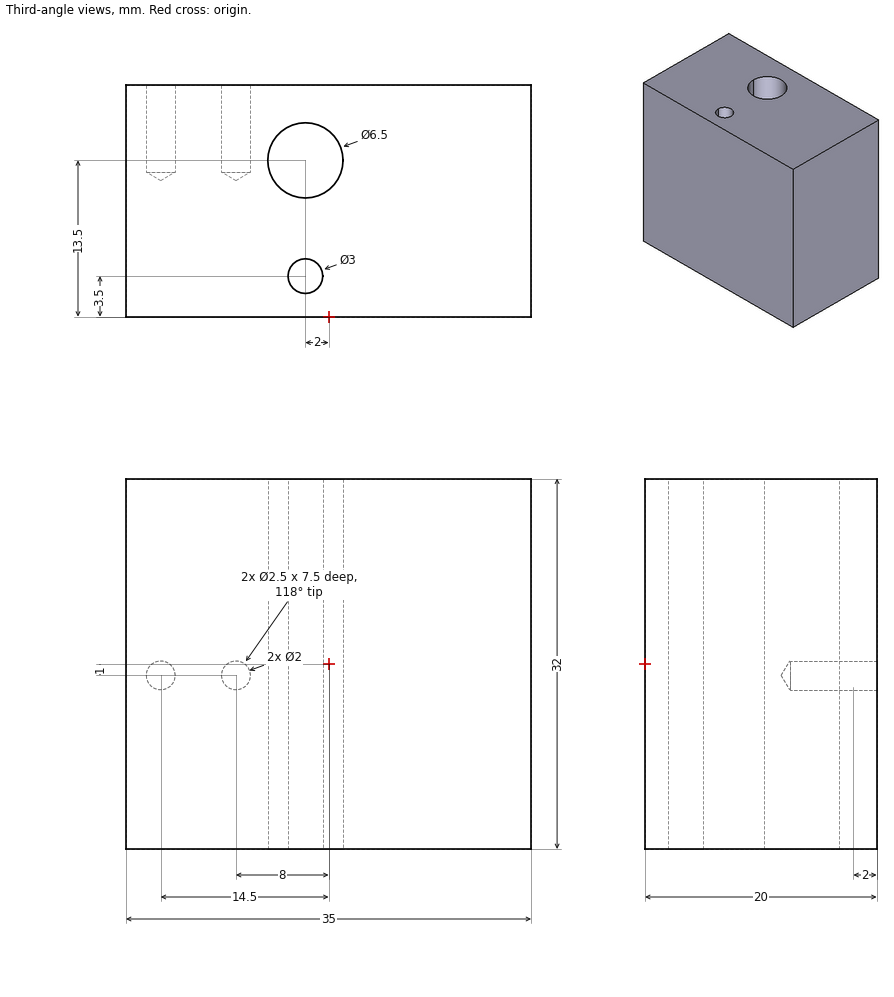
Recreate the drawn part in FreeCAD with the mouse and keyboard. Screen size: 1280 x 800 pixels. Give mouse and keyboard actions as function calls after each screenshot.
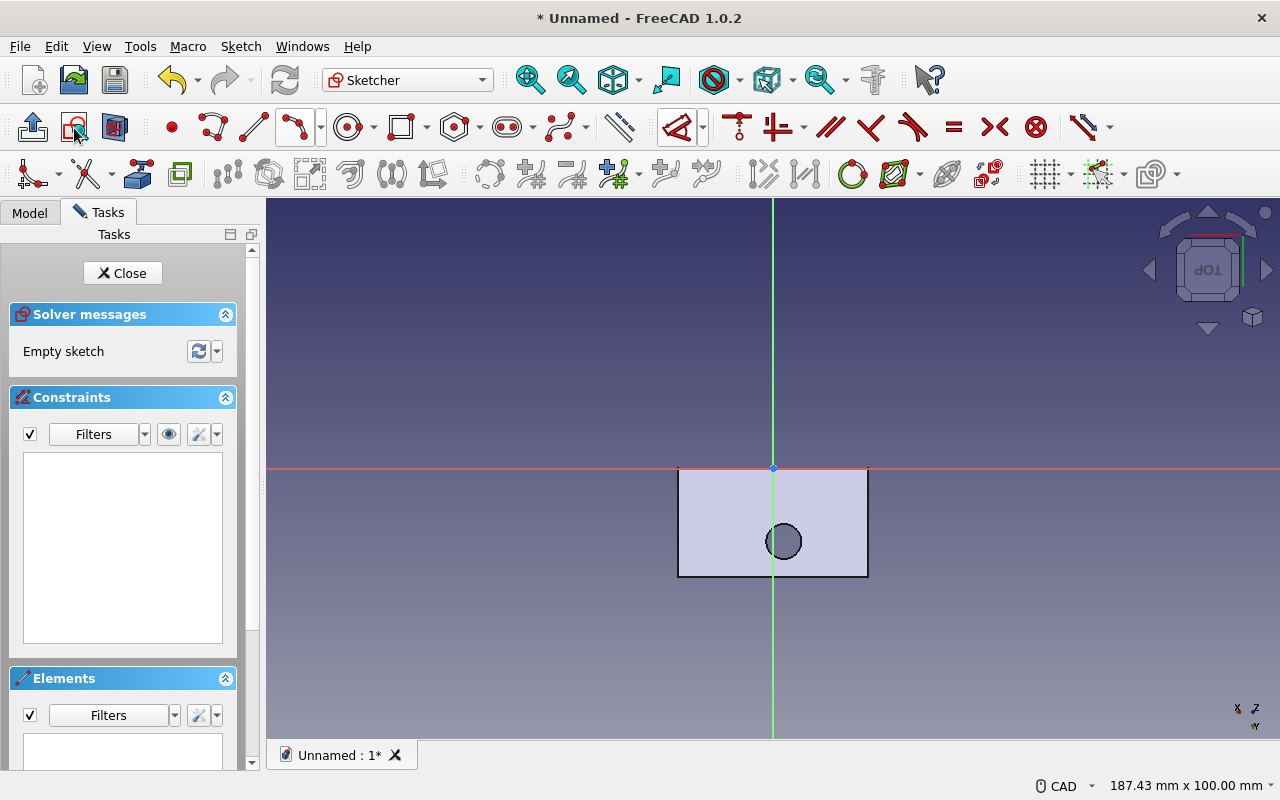
scroll(789, 483, up, 13)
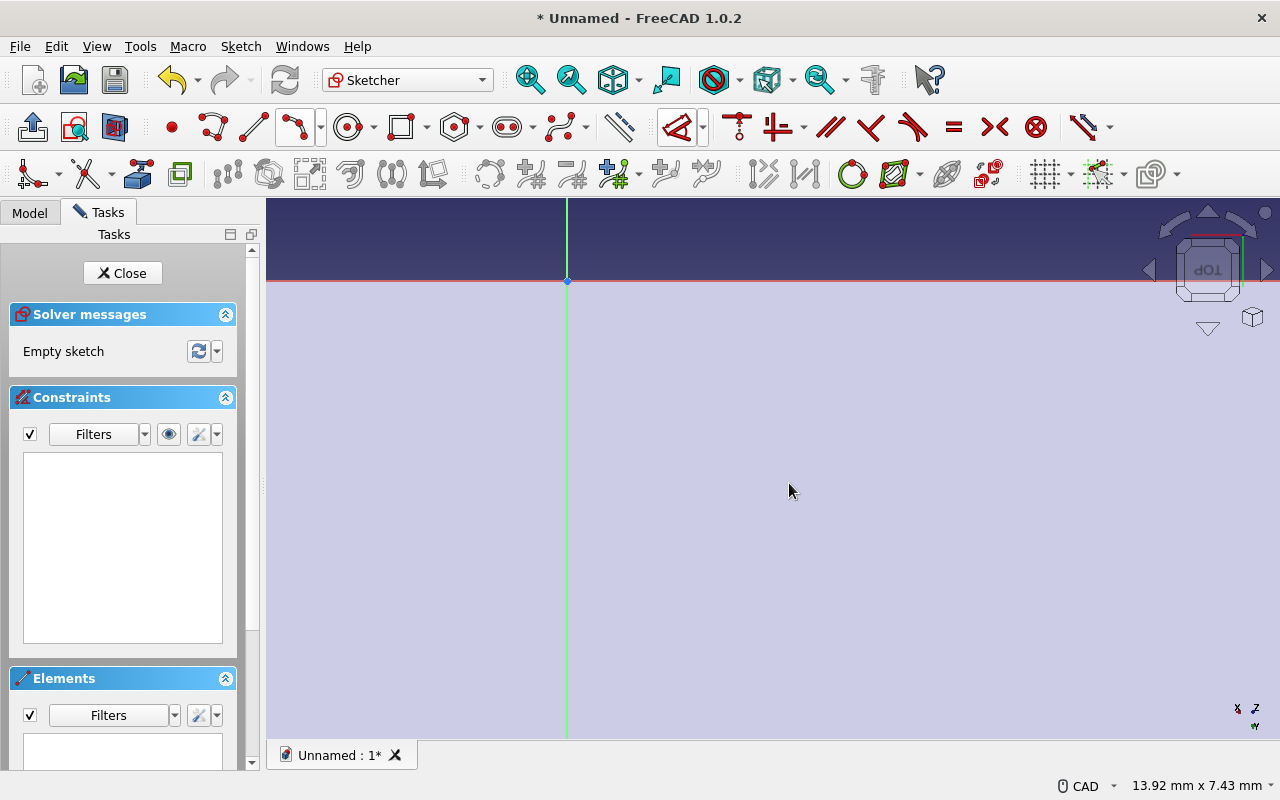
key(g)
key(c)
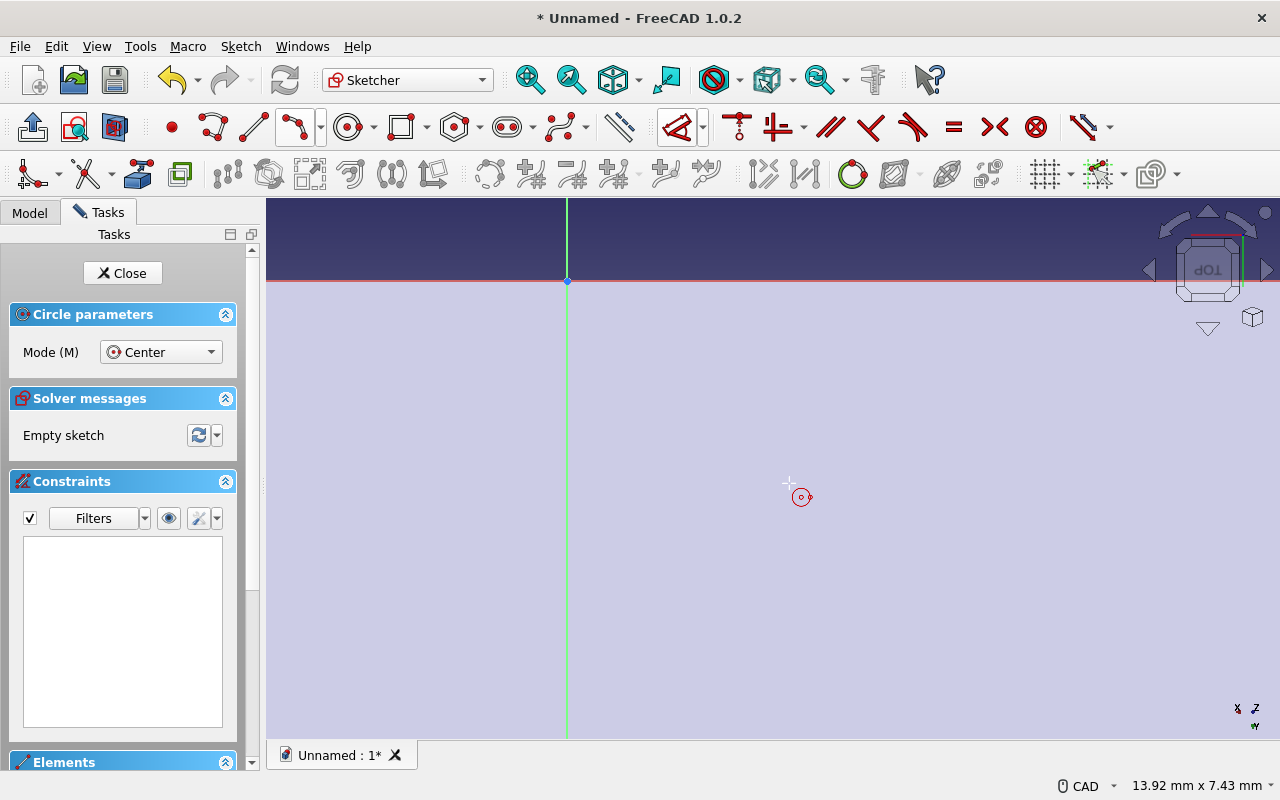
click(713, 536)
click(790, 459)
key(Escape)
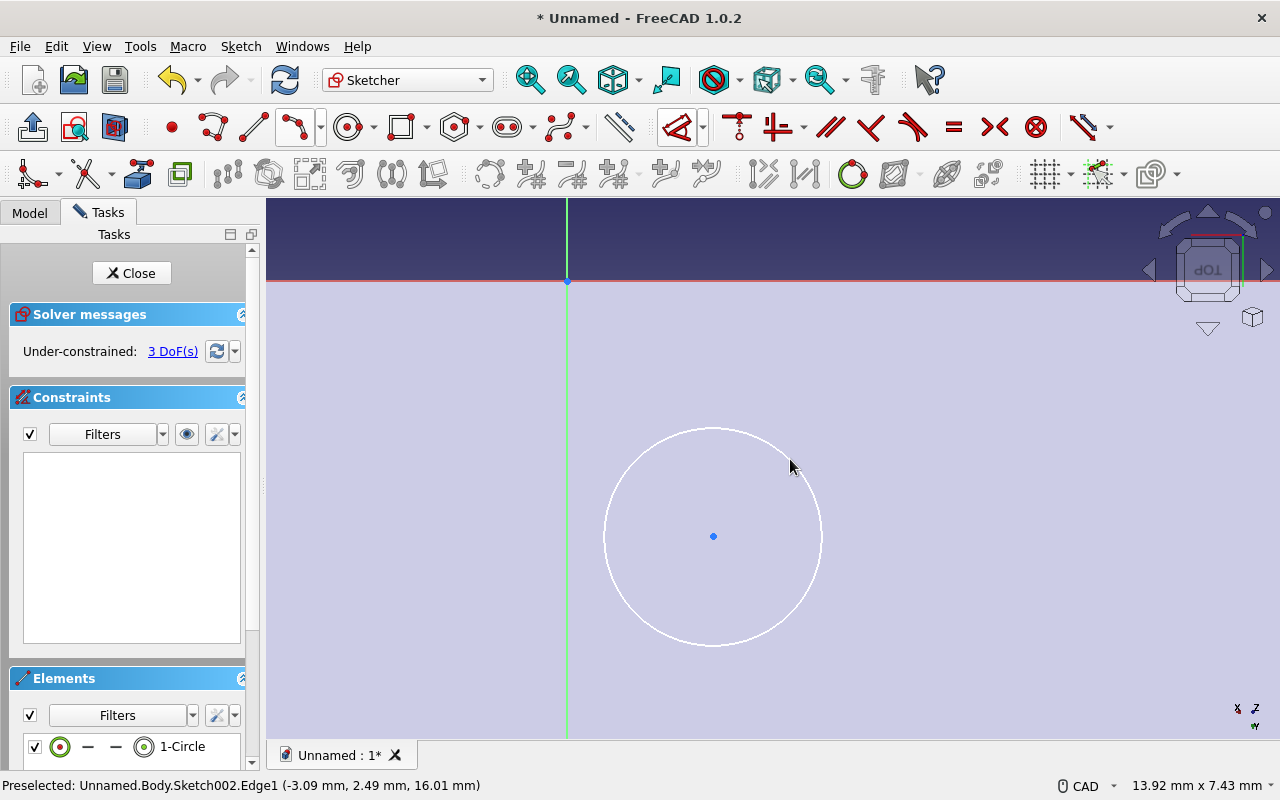
click(790, 460)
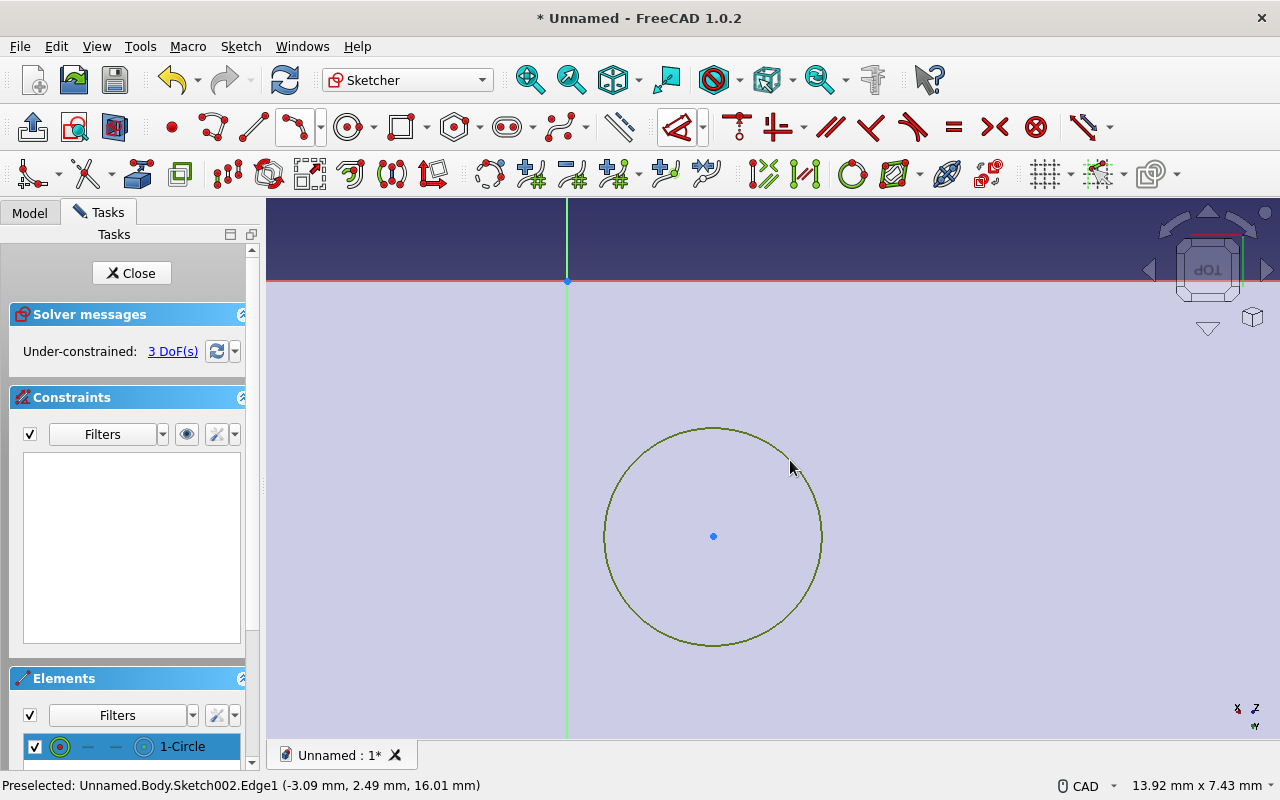
key(k)
key(o)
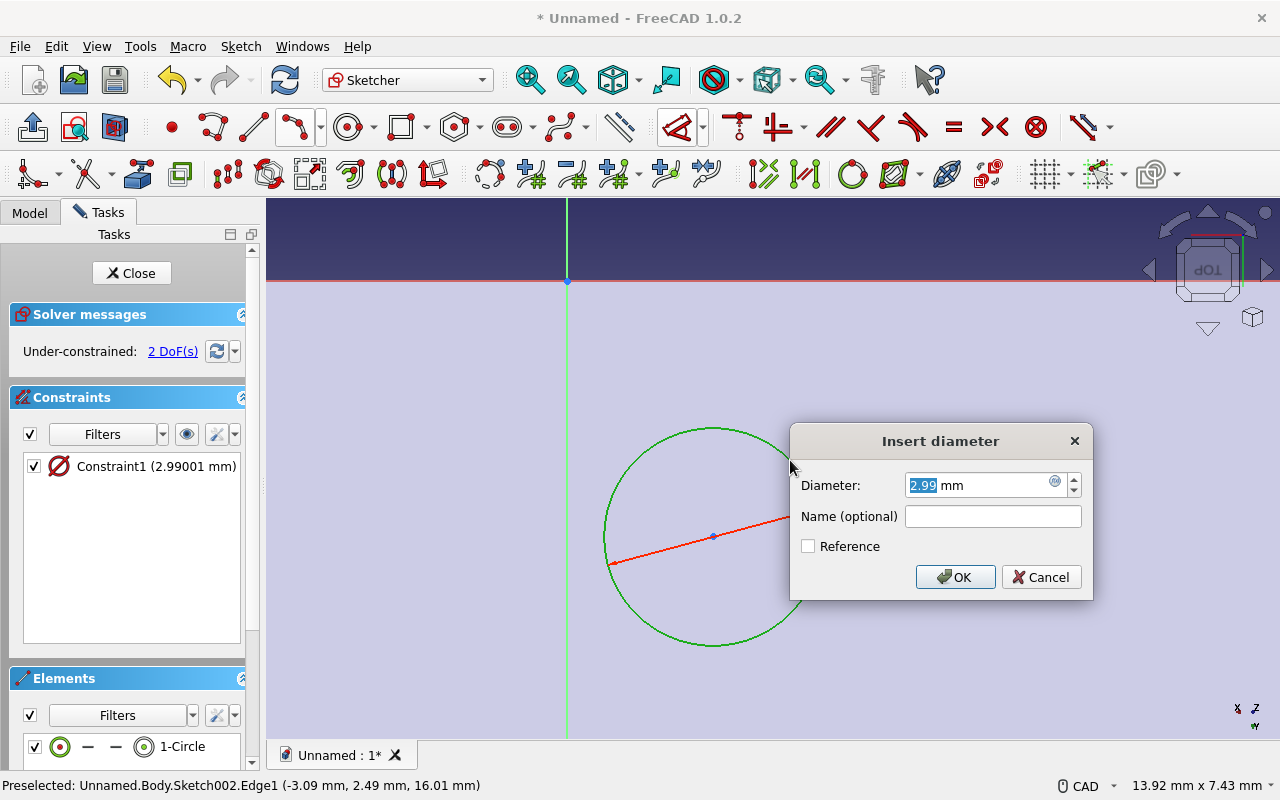
text(3)
key(Return)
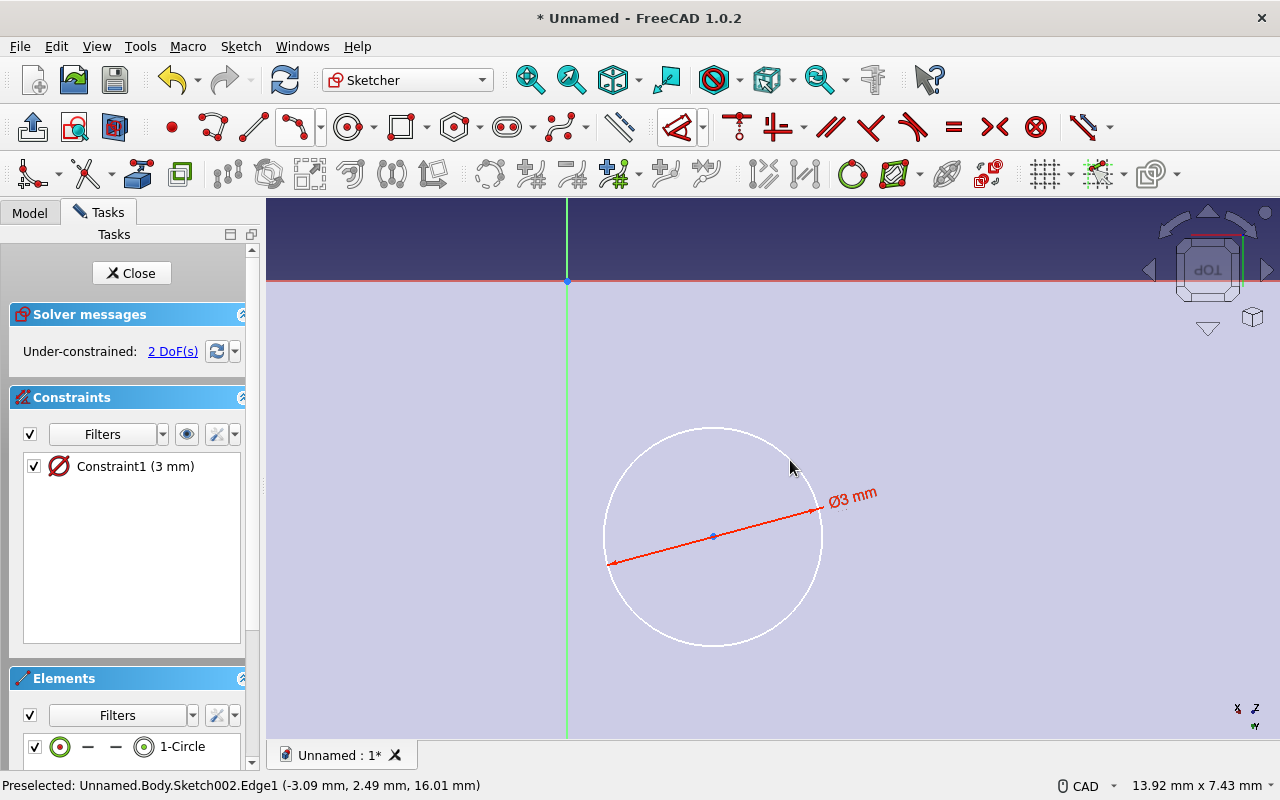
click(713, 537)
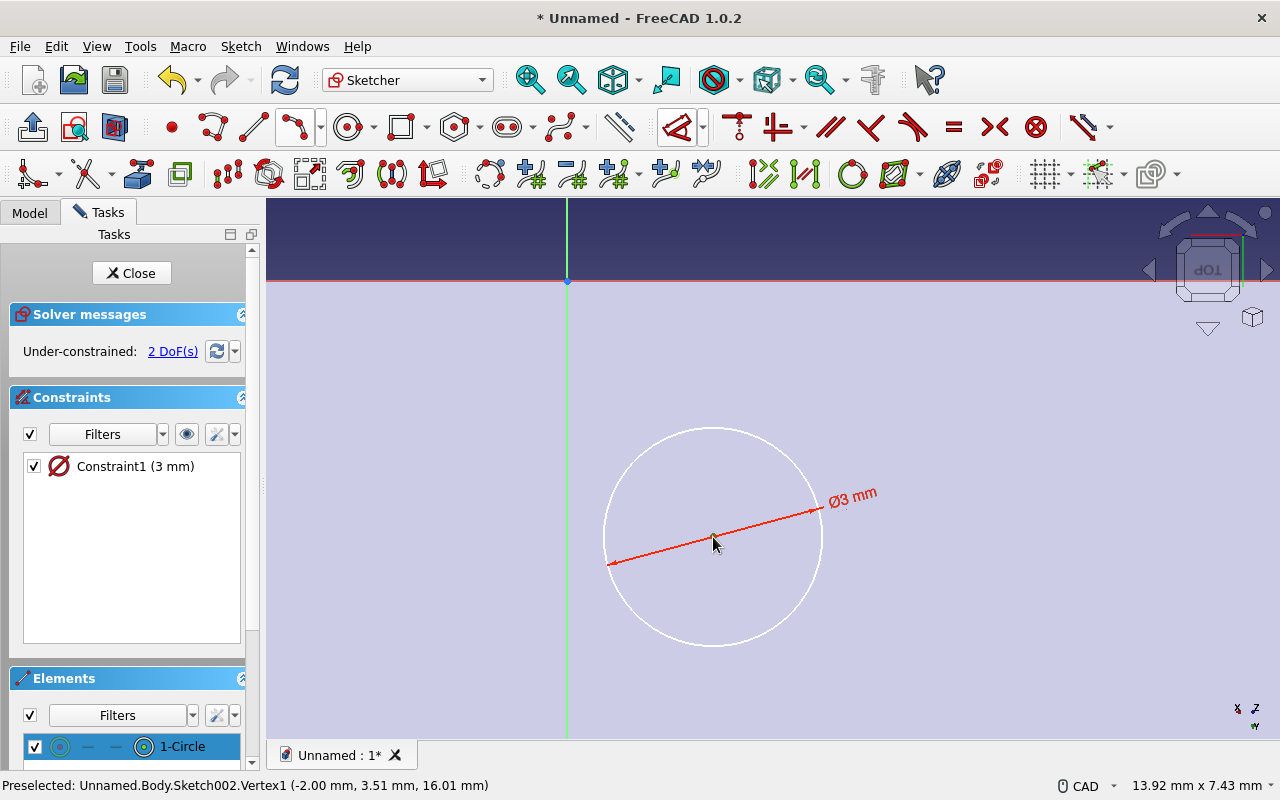
key(l)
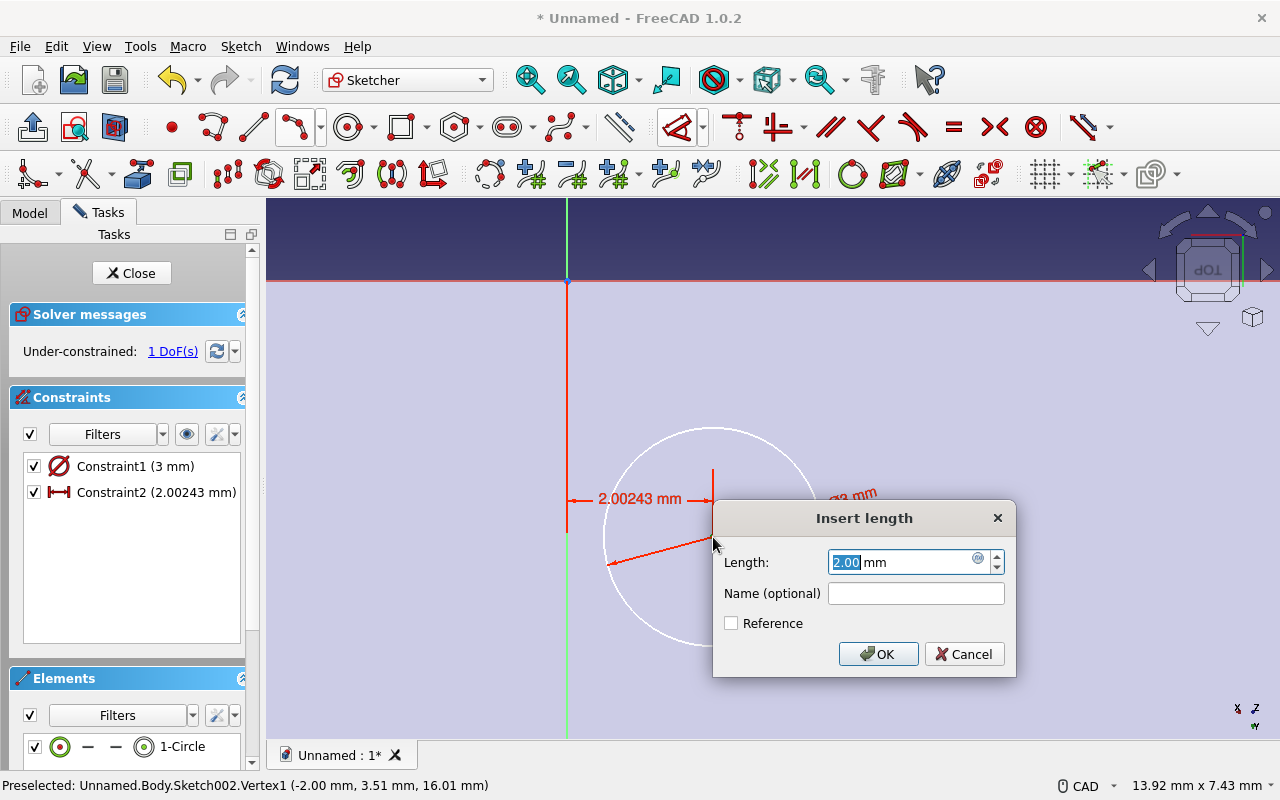
text(2)
key(Return)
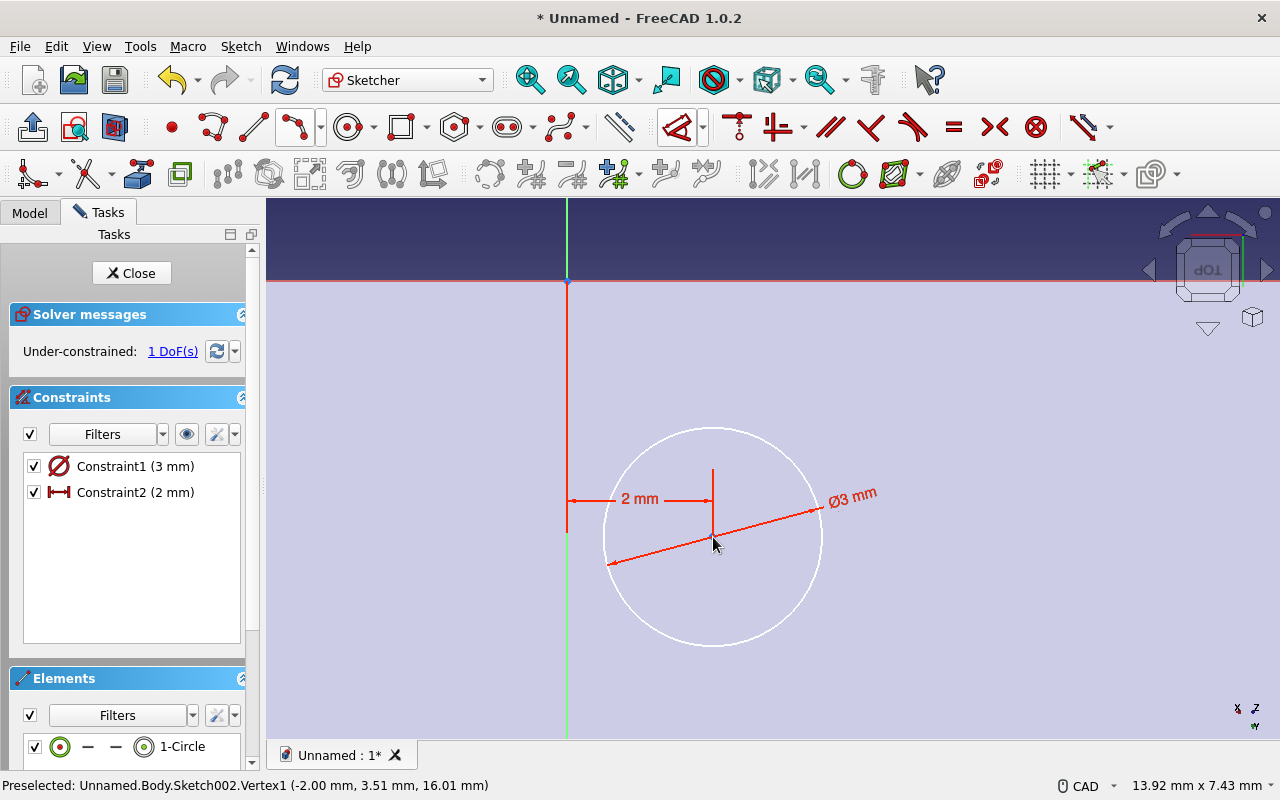
click(713, 537)